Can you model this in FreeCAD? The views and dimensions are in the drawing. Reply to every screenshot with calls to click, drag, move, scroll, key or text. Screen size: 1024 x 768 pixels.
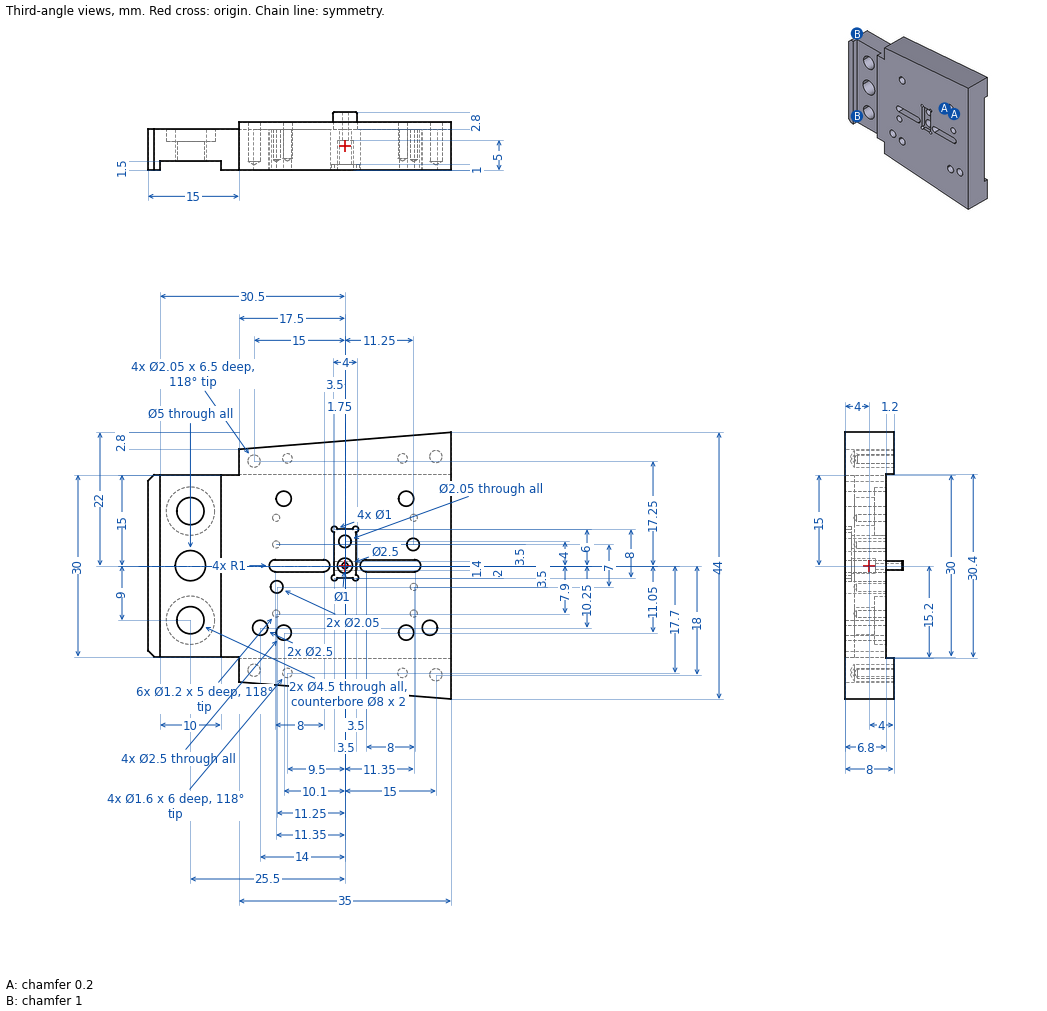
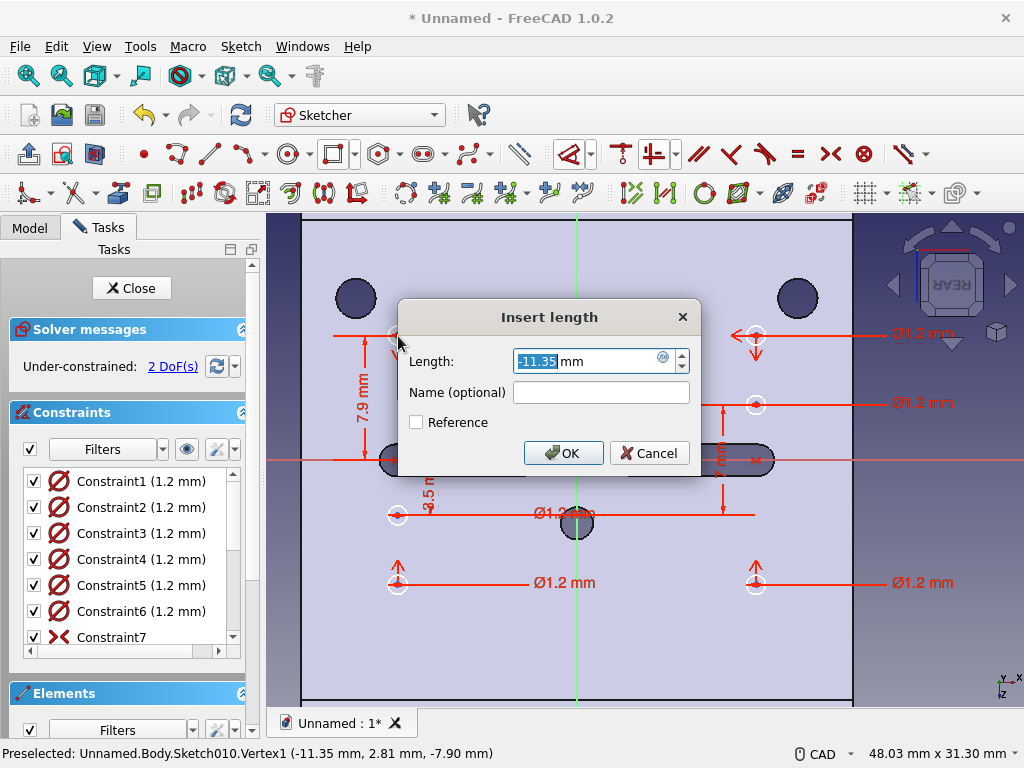
text(-11.35)
key(Return)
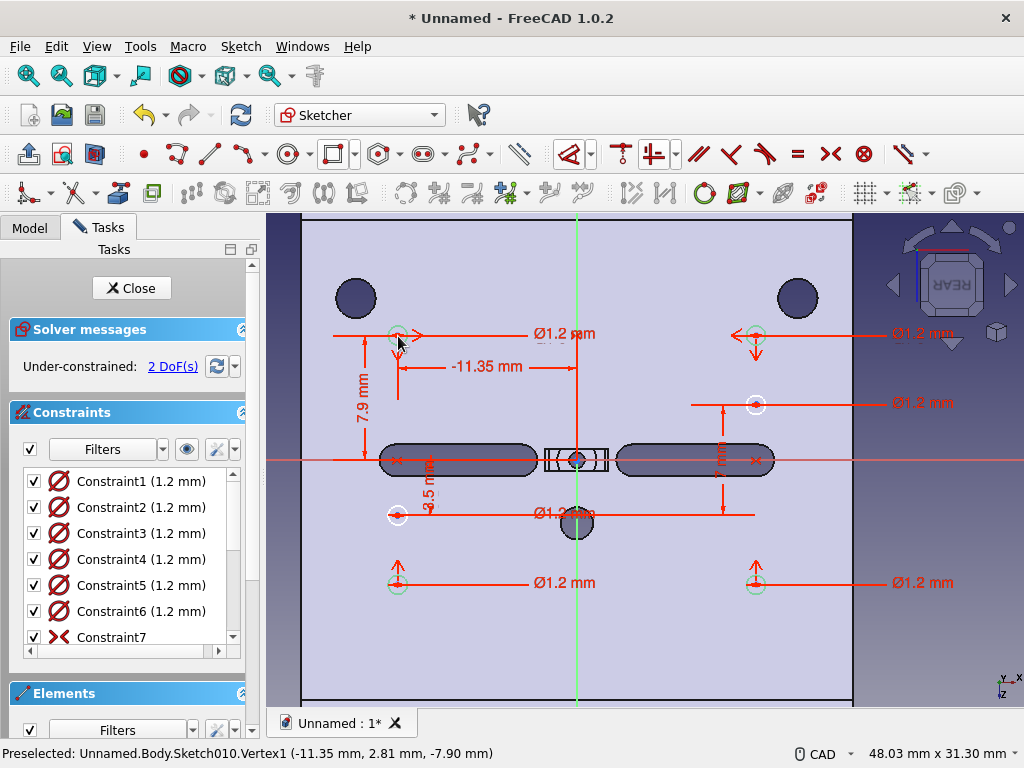
click(398, 515)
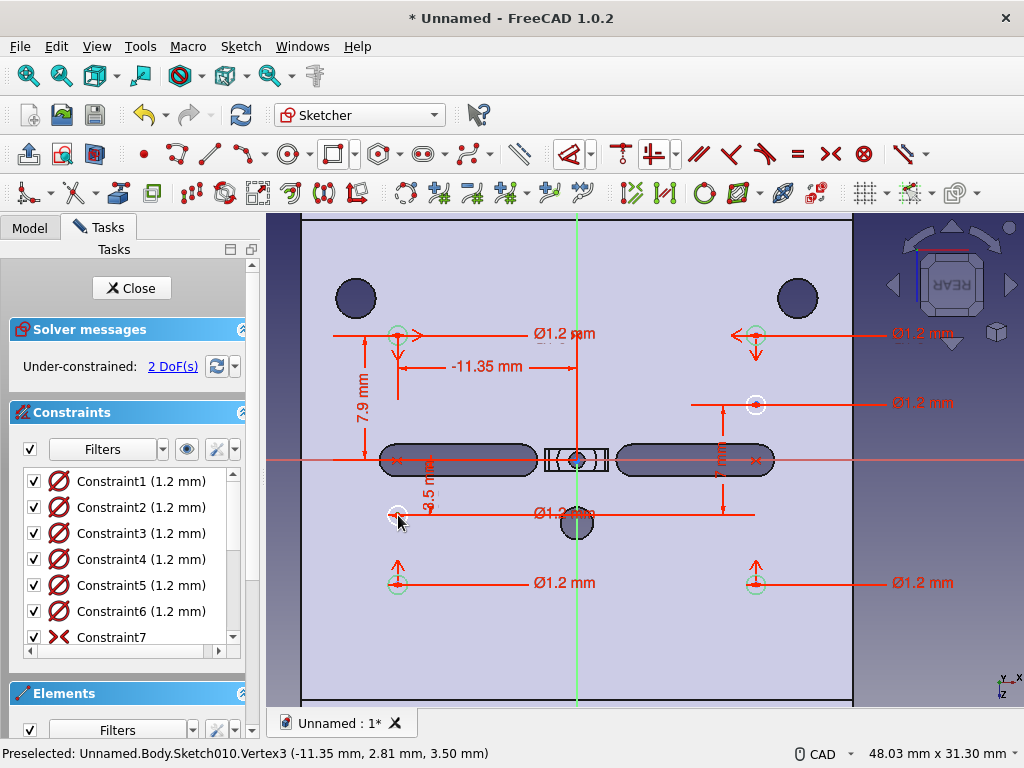
key(l)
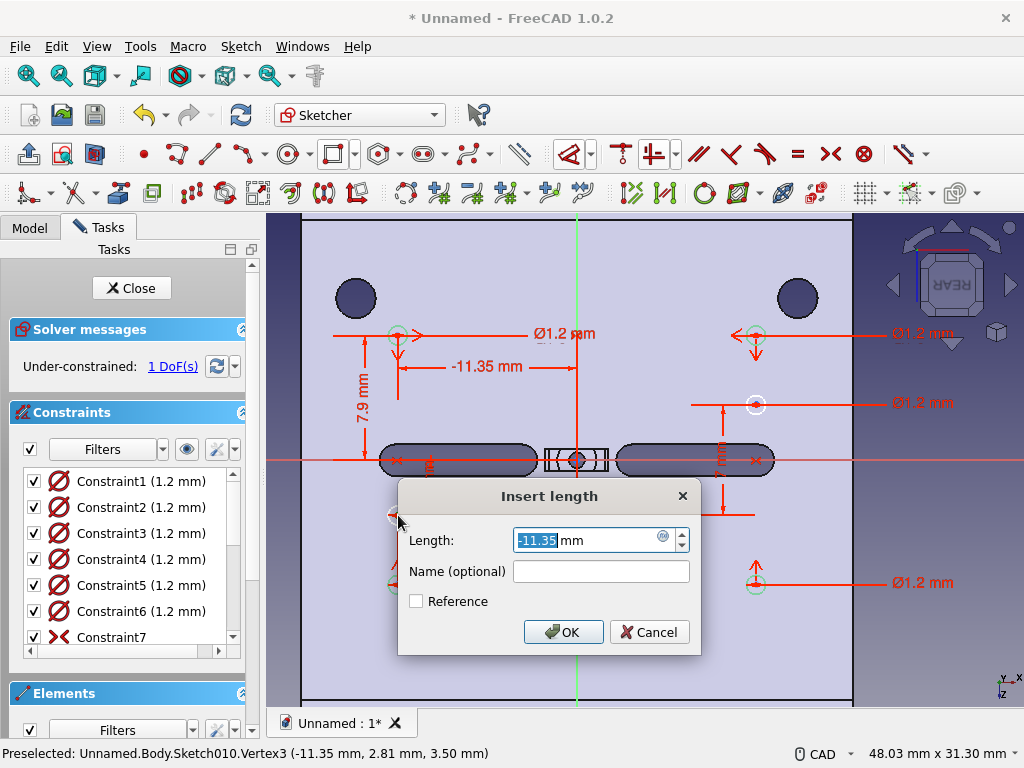
text(-11.35)
key(Return)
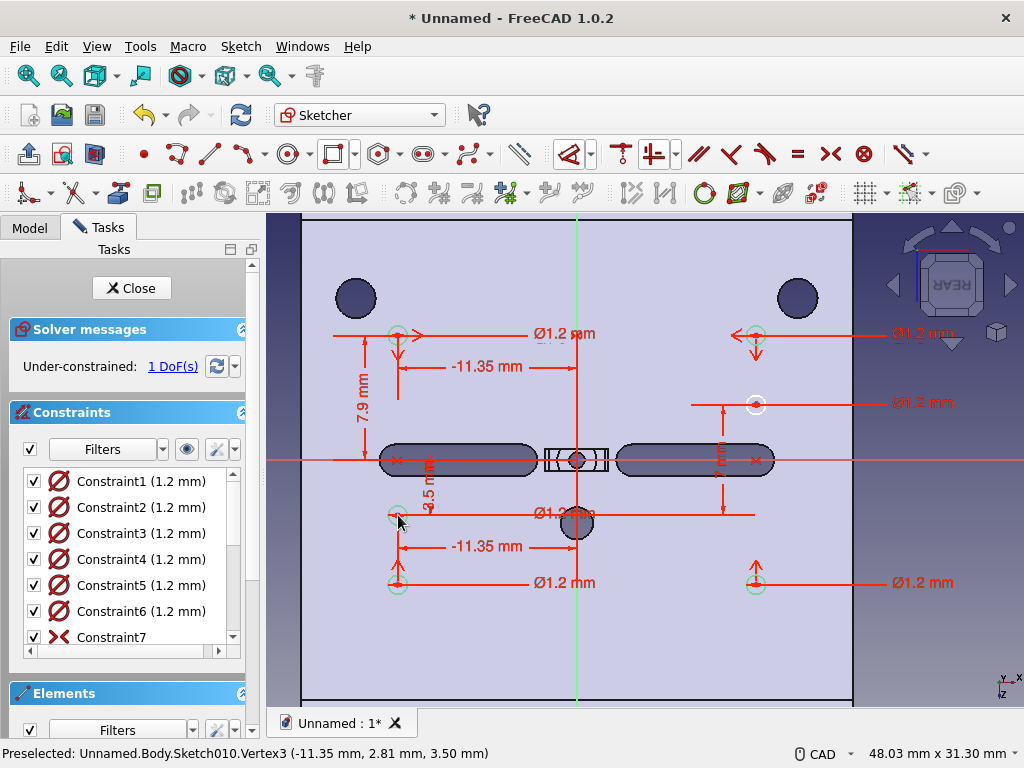
click(756, 405)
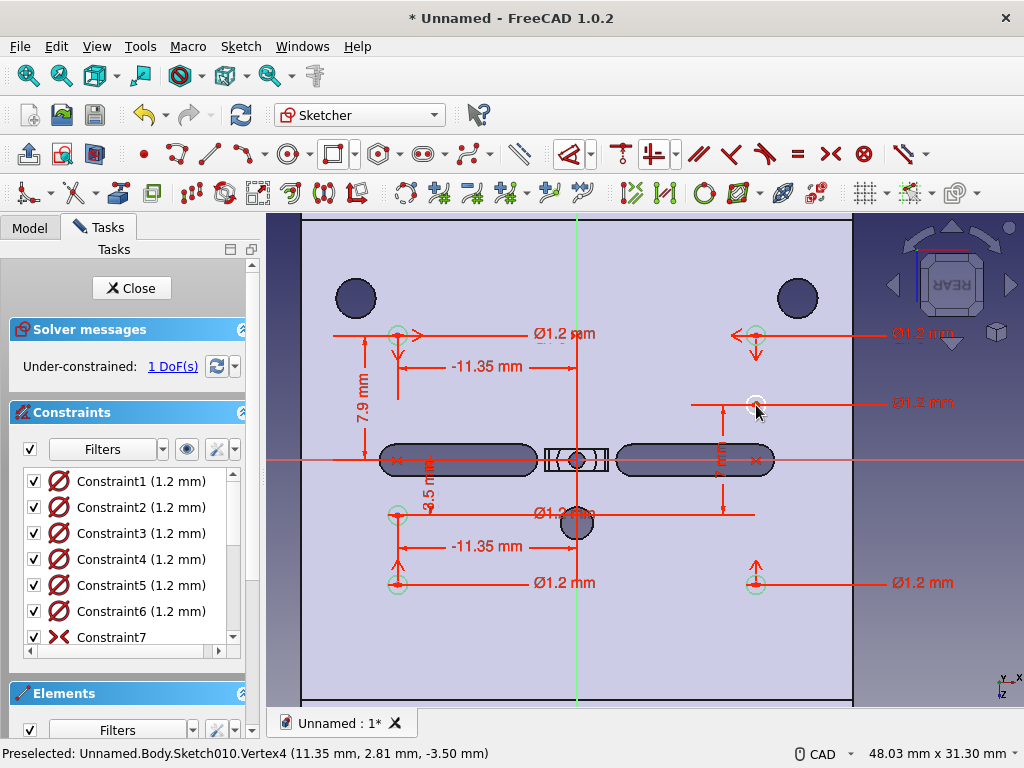
key(l)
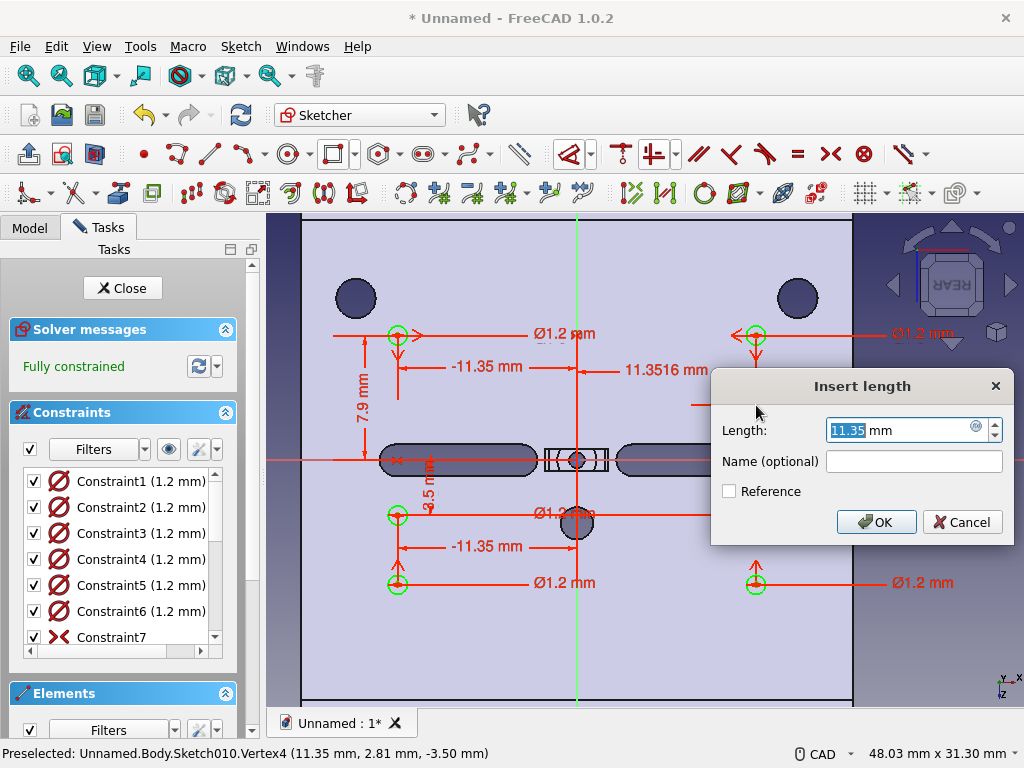
text(11.35)
key(Return)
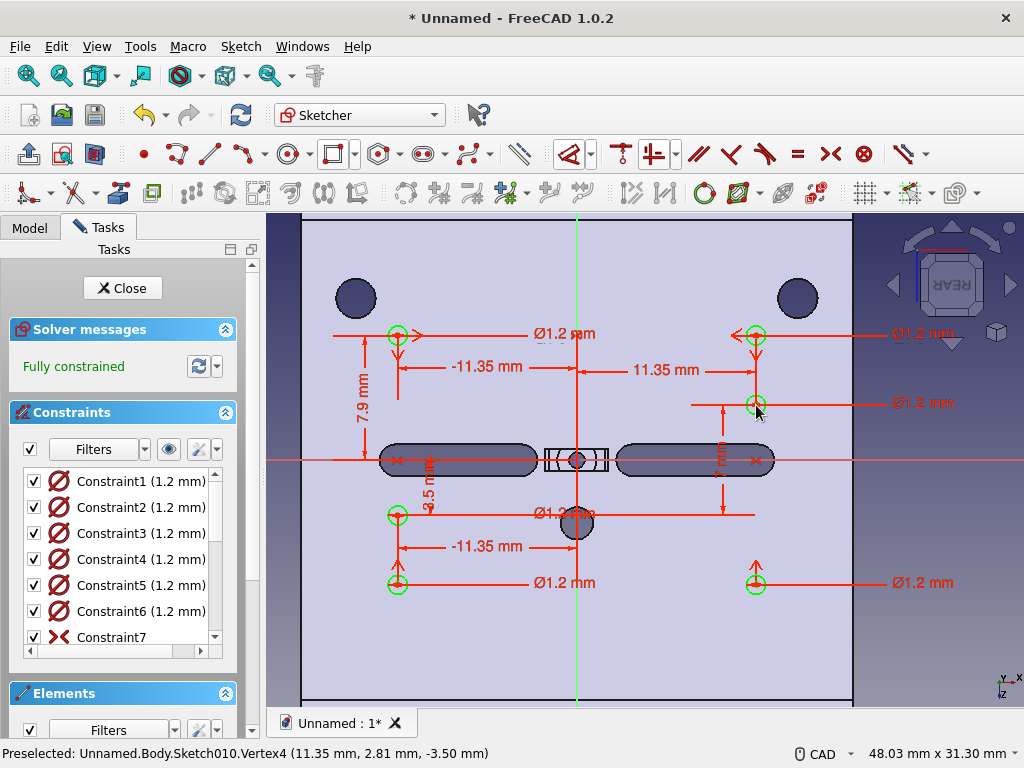
click(123, 288)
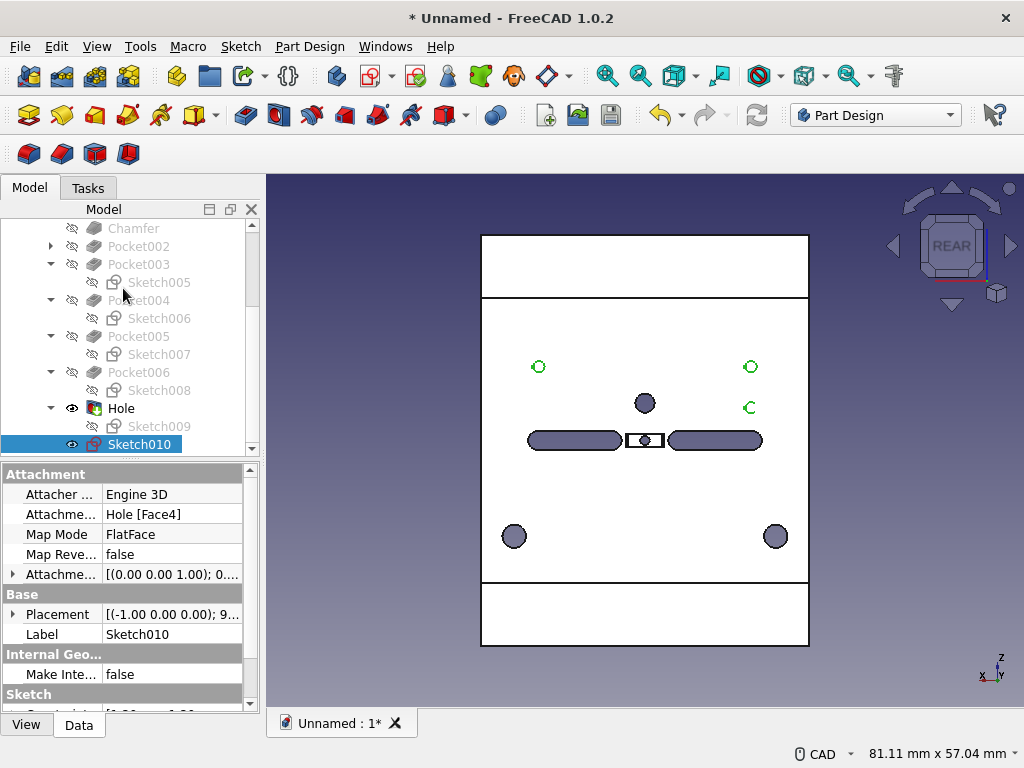
click(279, 116)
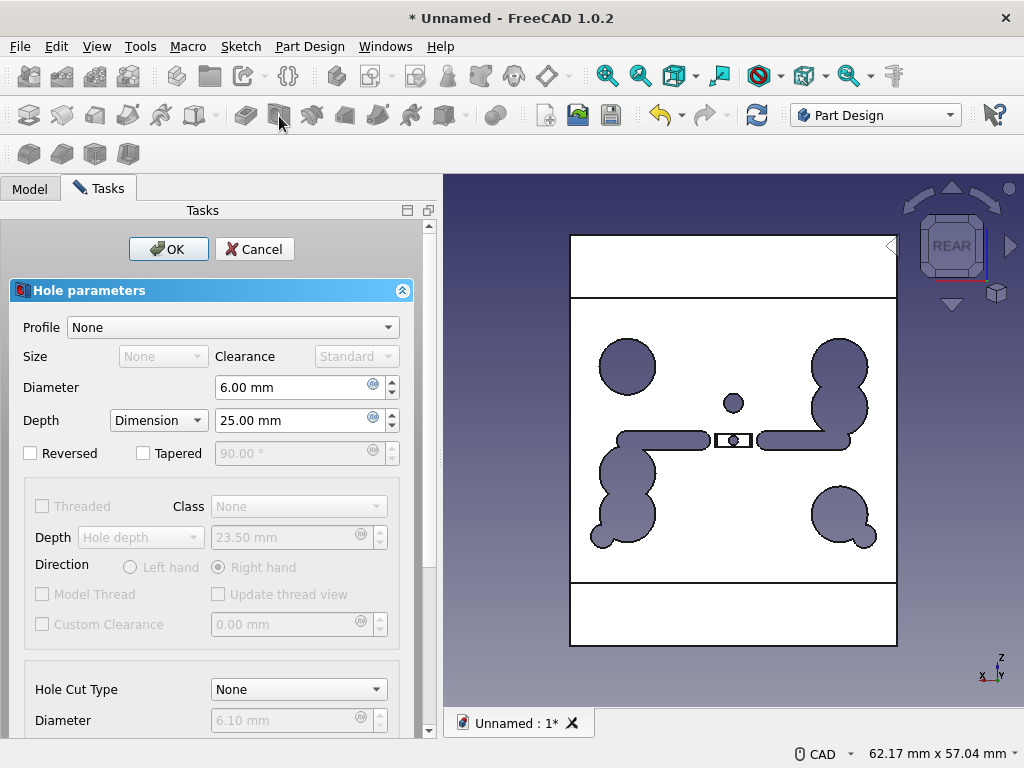
triple_click(300, 388)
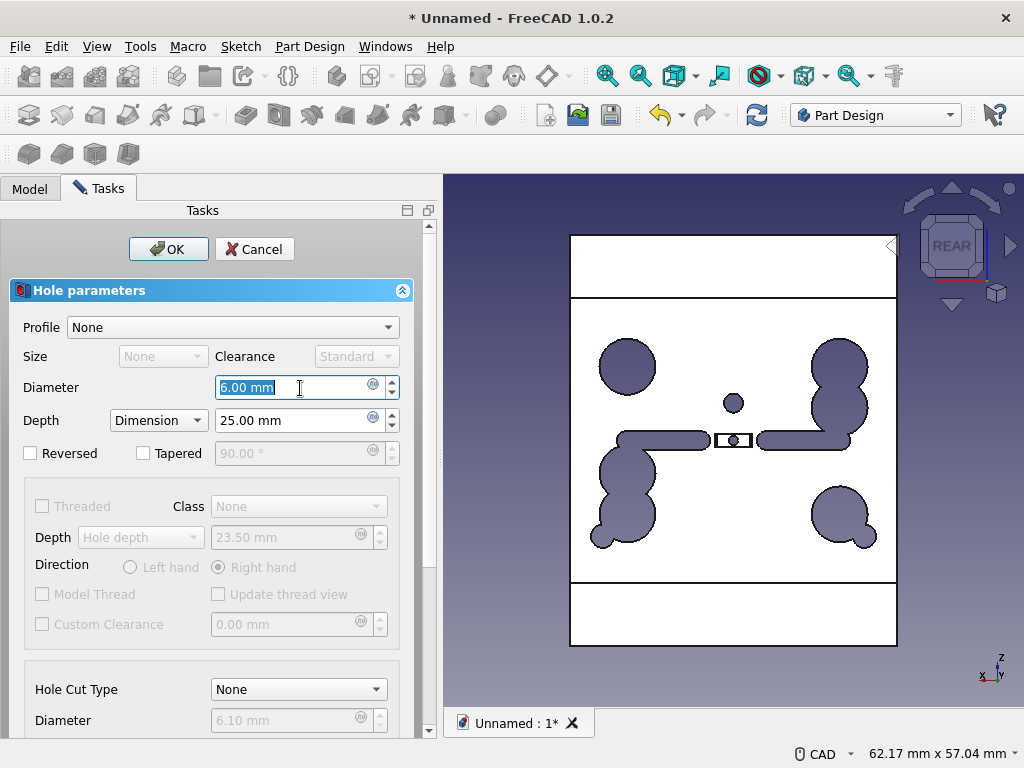
text(1.2)
key(Tab)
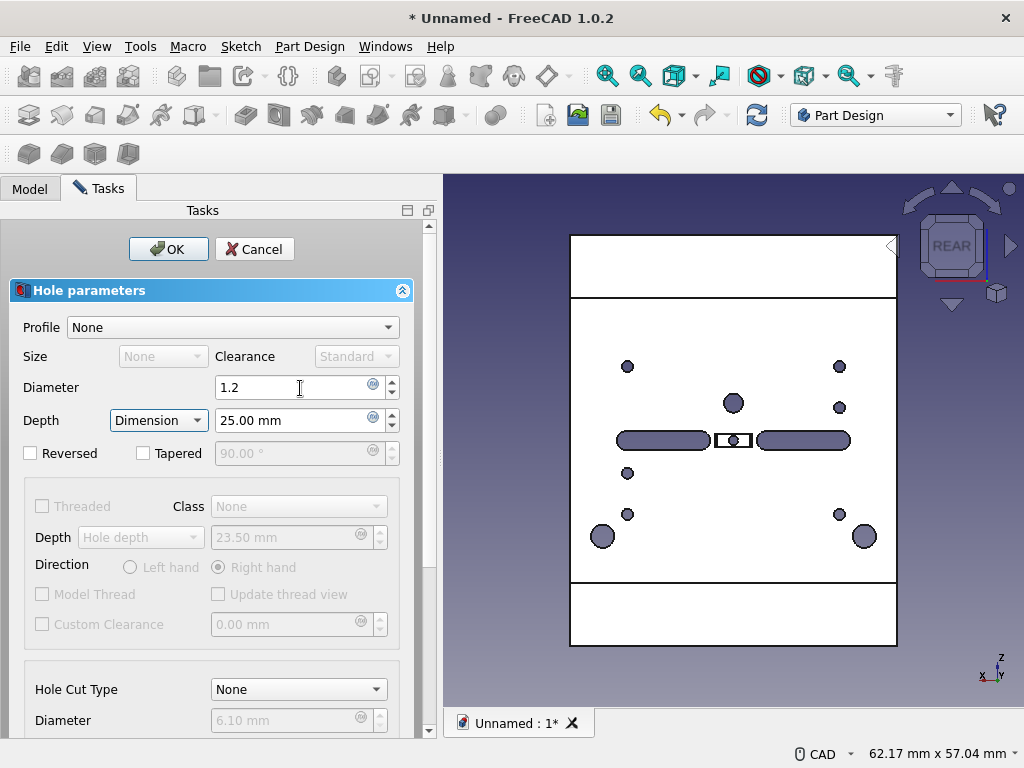
triple_click(300, 420)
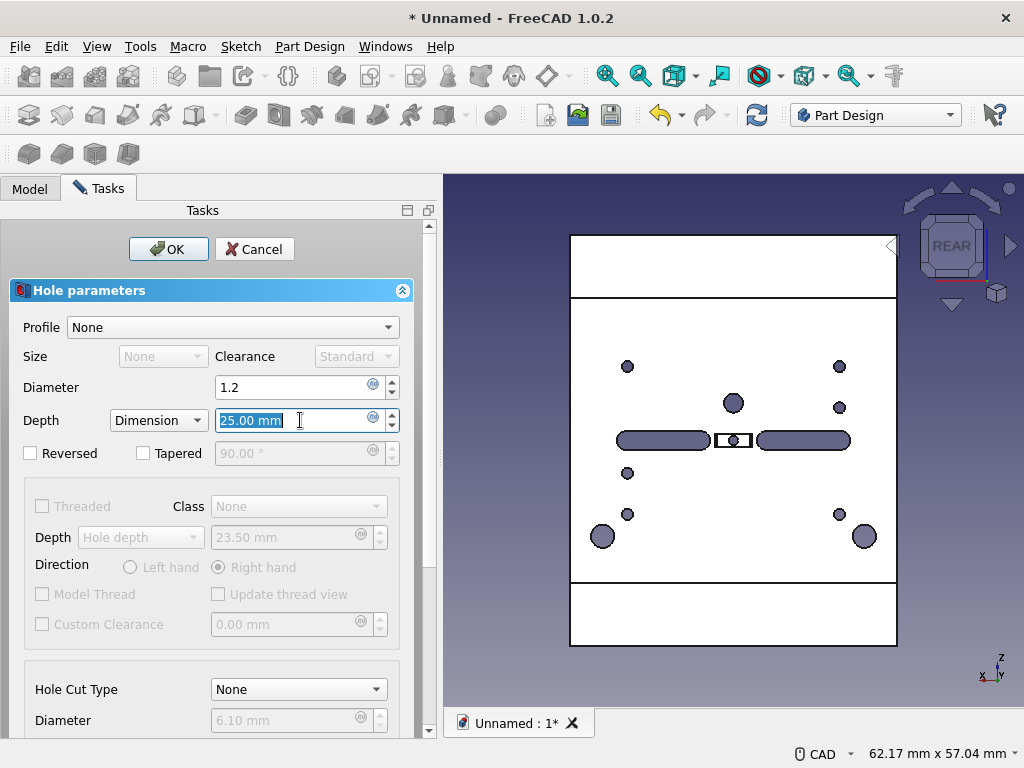
text(5)
key(Tab)